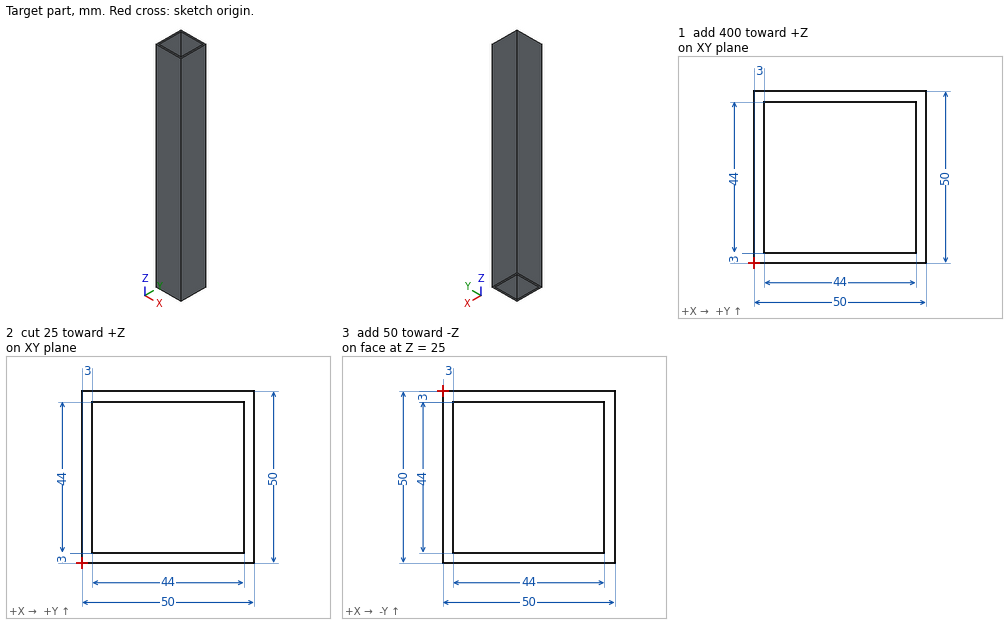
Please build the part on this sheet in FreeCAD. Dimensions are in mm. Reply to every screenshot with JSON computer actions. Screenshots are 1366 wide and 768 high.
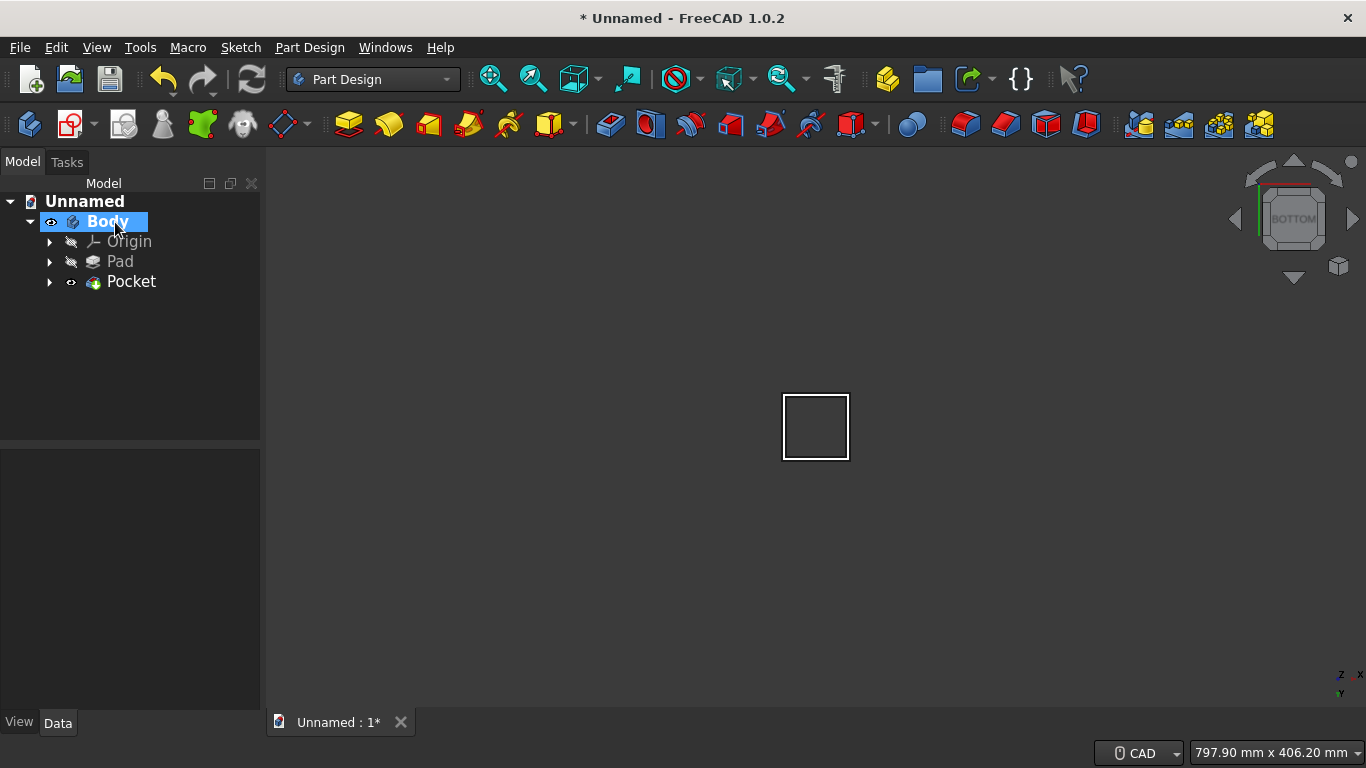
{"action": "left_click", "coordinate": [494, 80]}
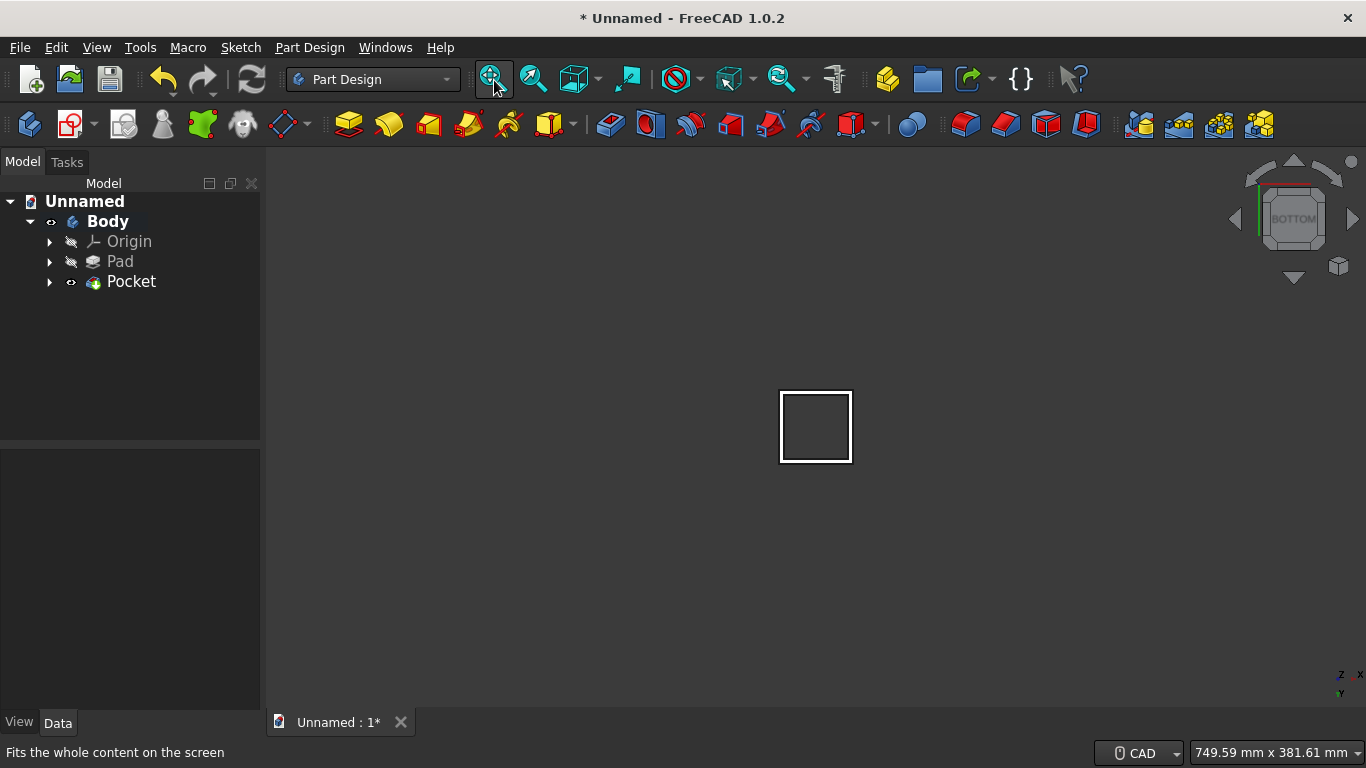
{"action": "scroll", "coordinate": [851, 415], "scroll_direction": "up", "scroll_amount": 11}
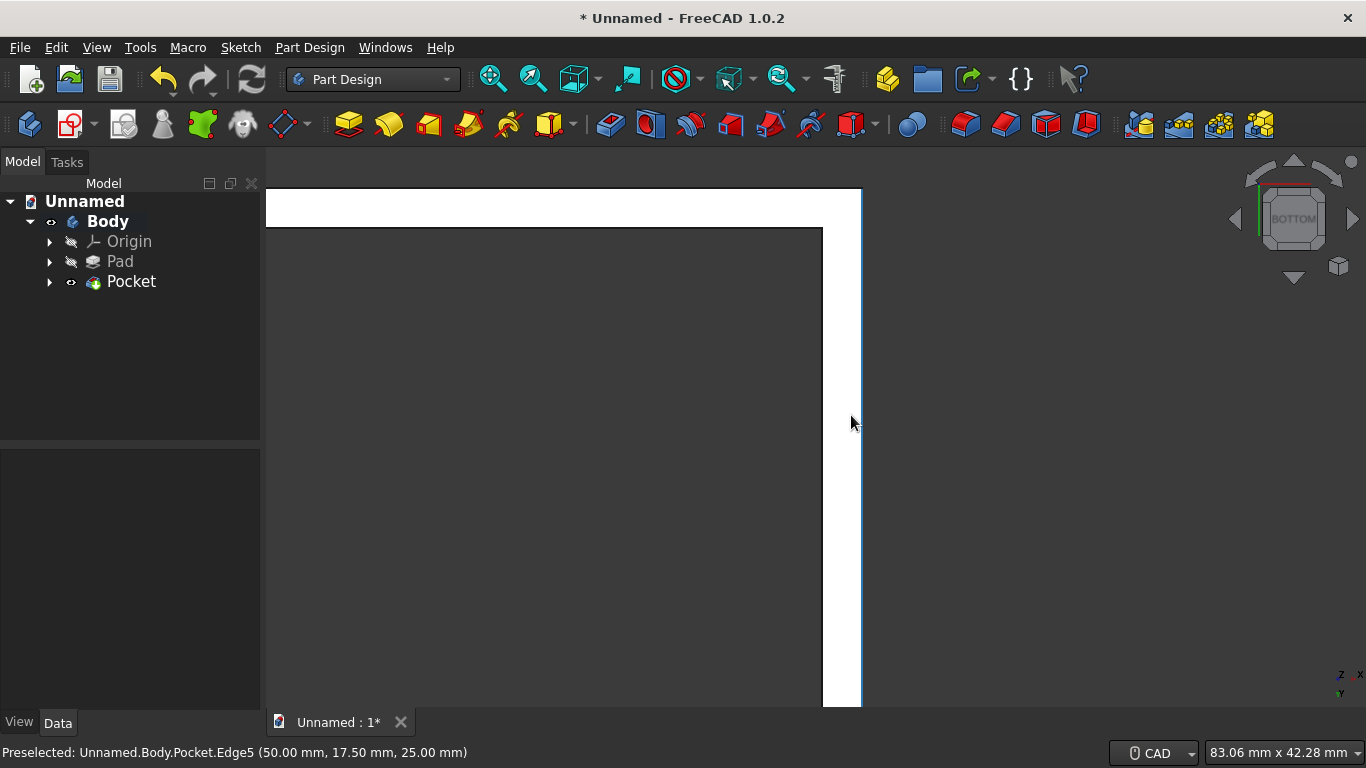
{"action": "left_click", "coordinate": [849, 421]}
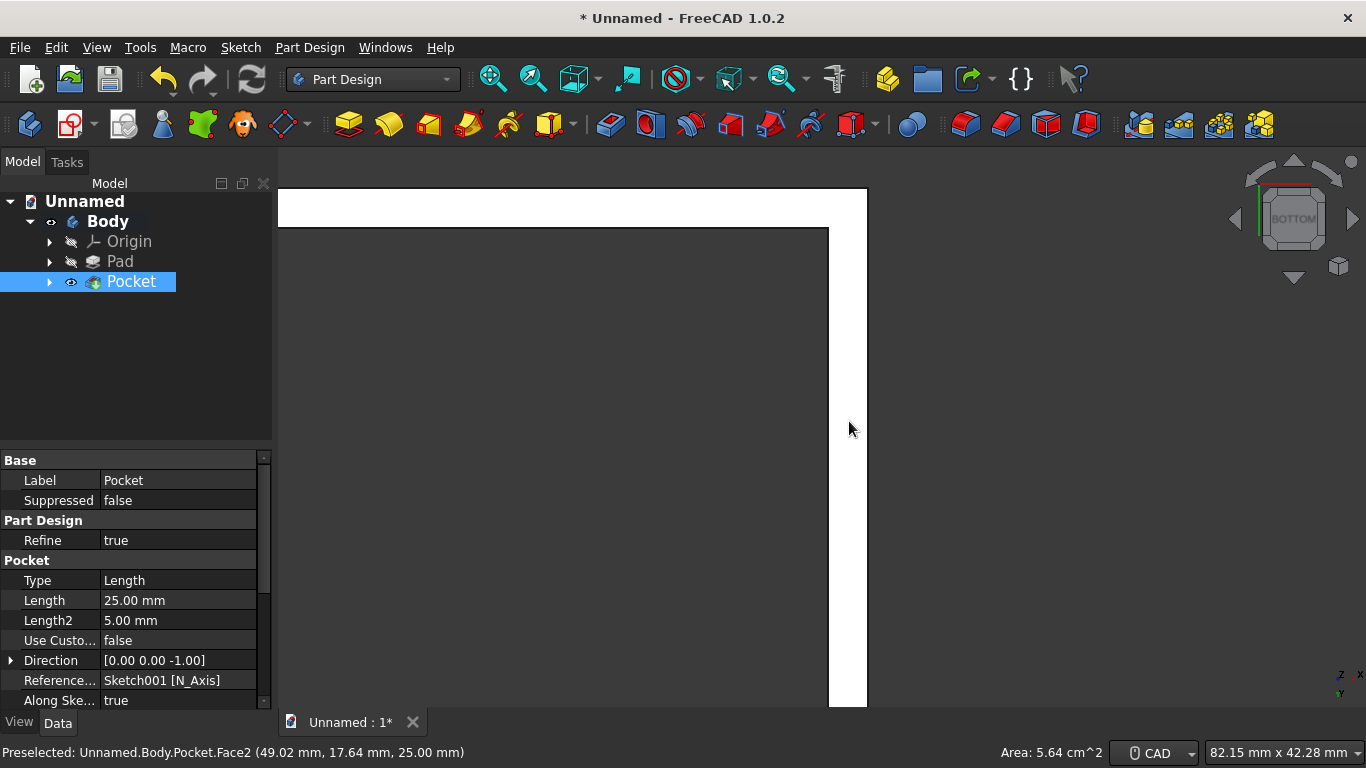
{"action": "left_click", "coordinate": [70, 124]}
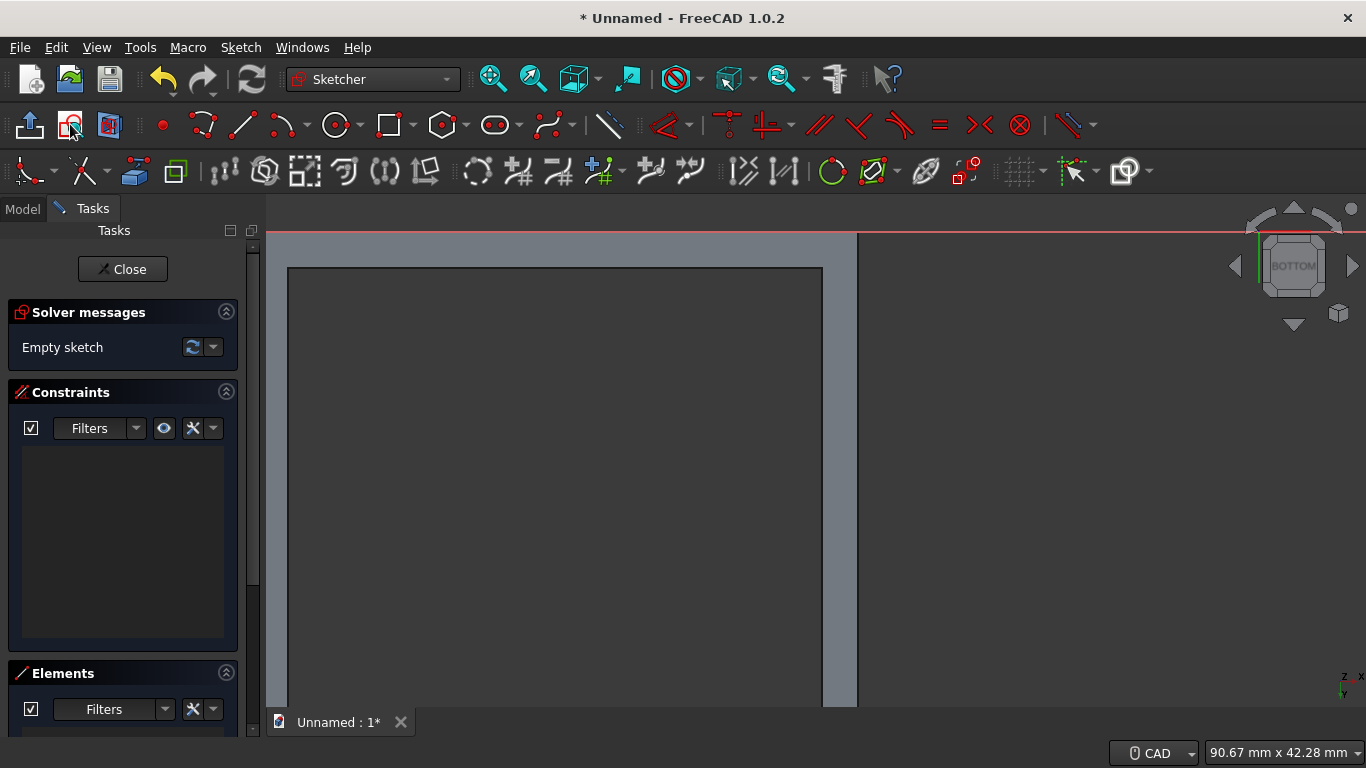
{"action": "scroll", "coordinate": [982, 347], "scroll_direction": "down", "scroll_amount": 3}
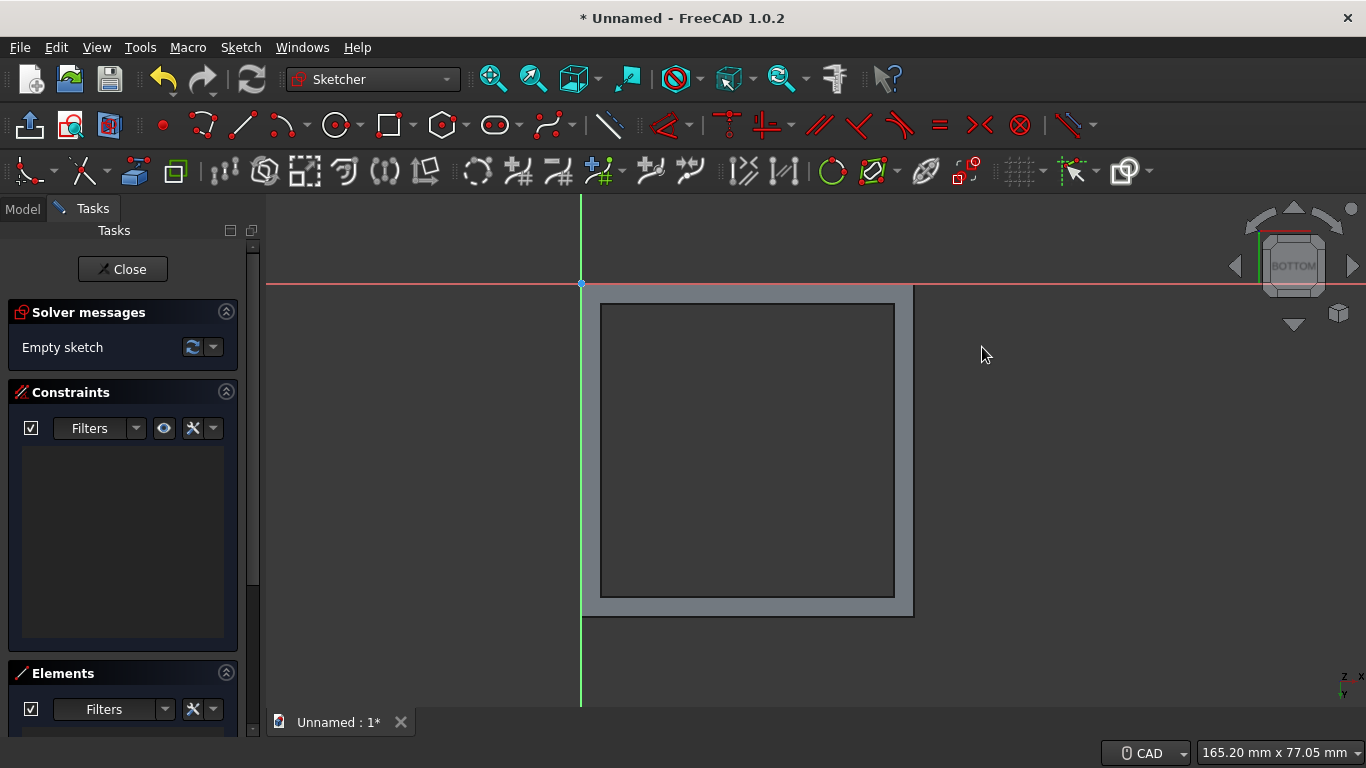
{"action": "left_click", "coordinate": [390, 126]}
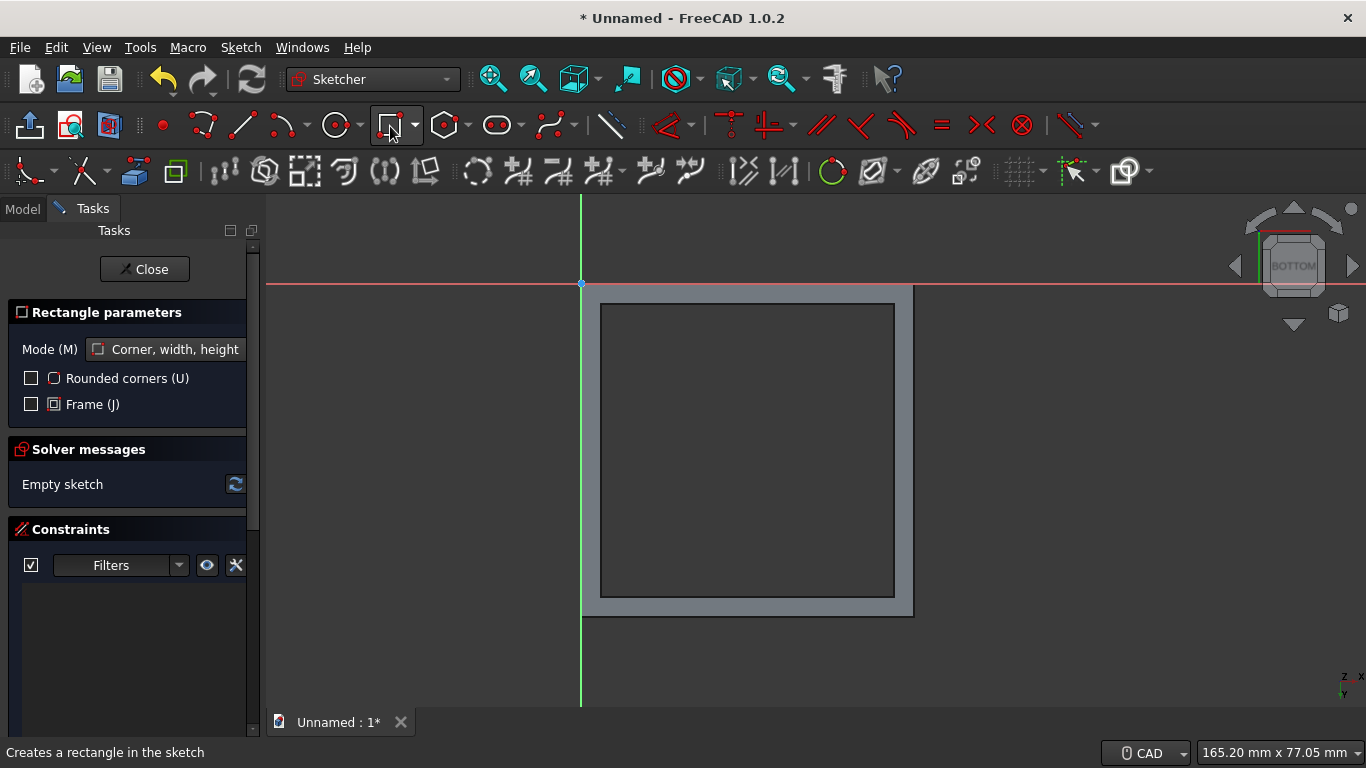
{"action": "left_click", "coordinate": [581, 284]}
{"action": "left_click", "coordinate": [914, 617]}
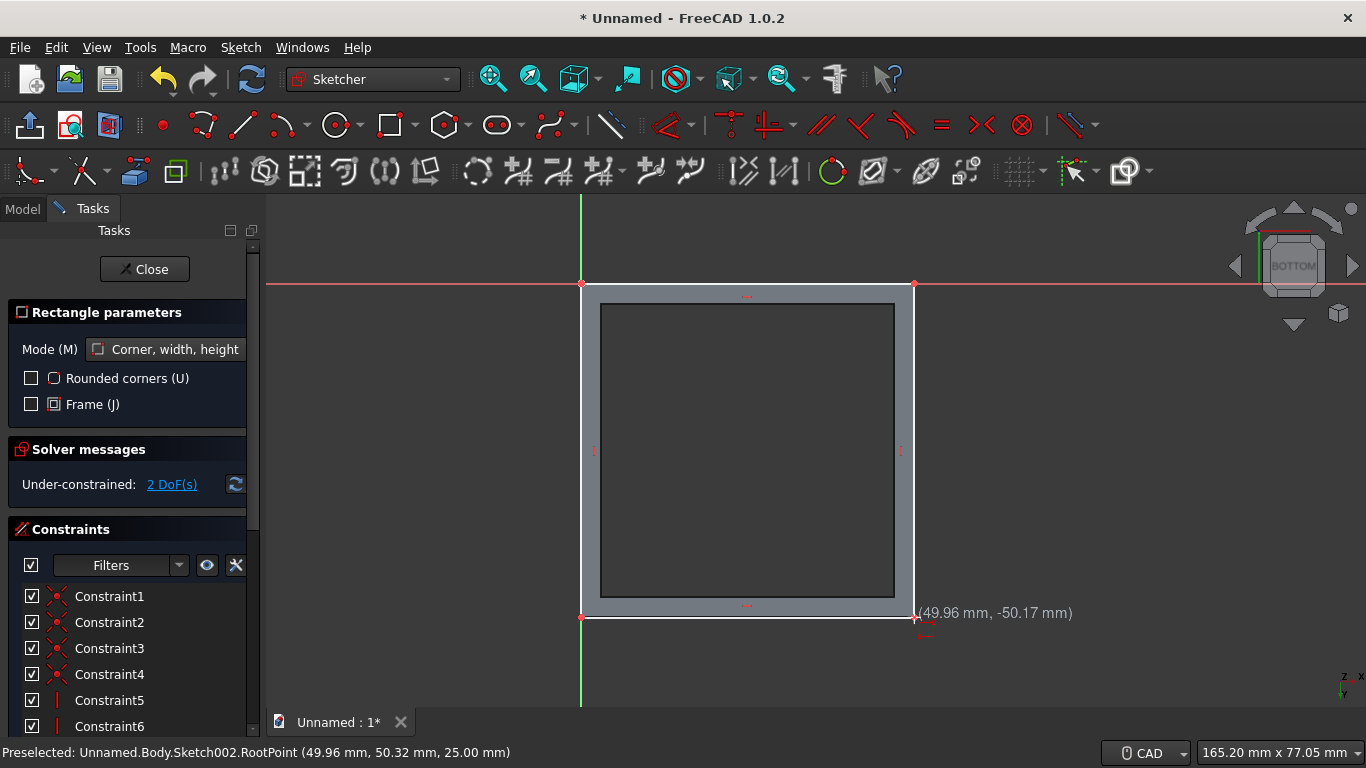
{"action": "left_click", "coordinate": [601, 304]}
{"action": "left_click", "coordinate": [894, 597]}
{"action": "key", "text": "Escape"}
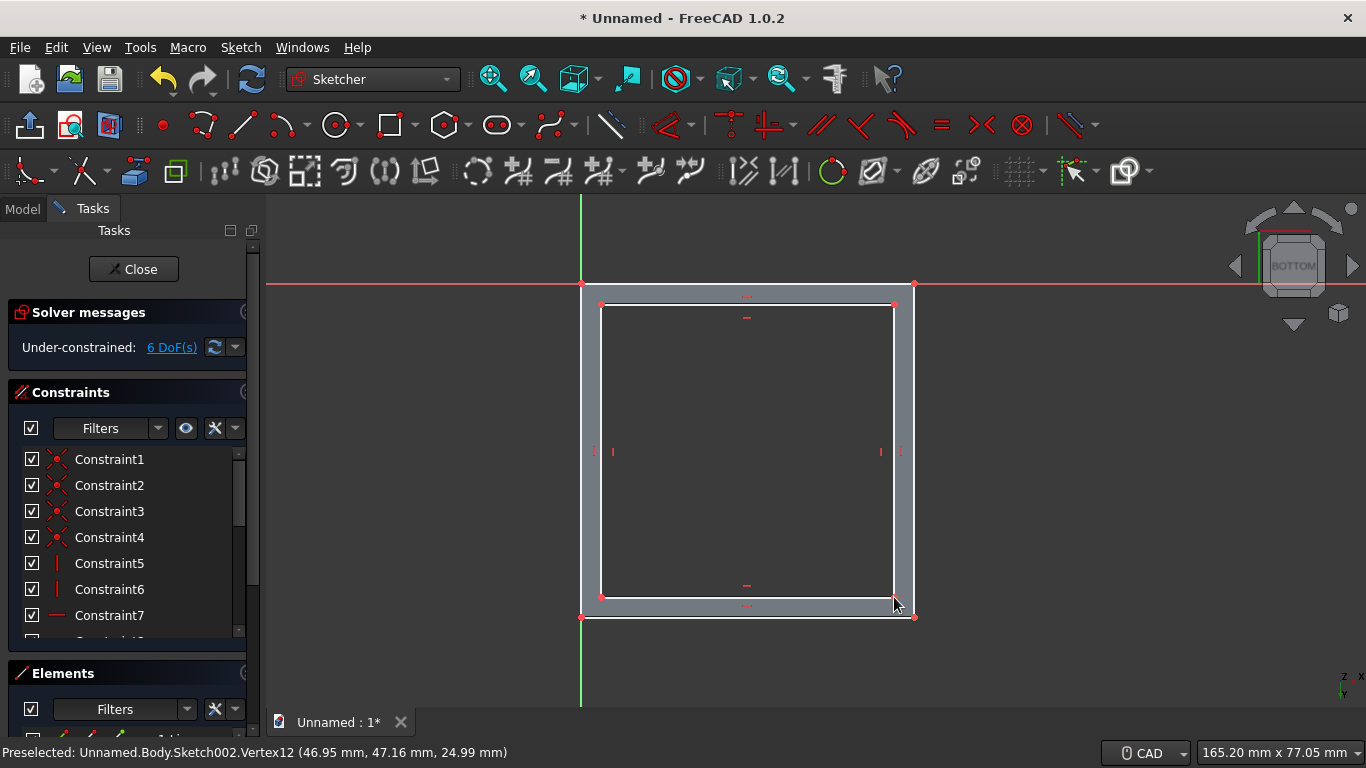
{"action": "left_click", "coordinate": [666, 126]}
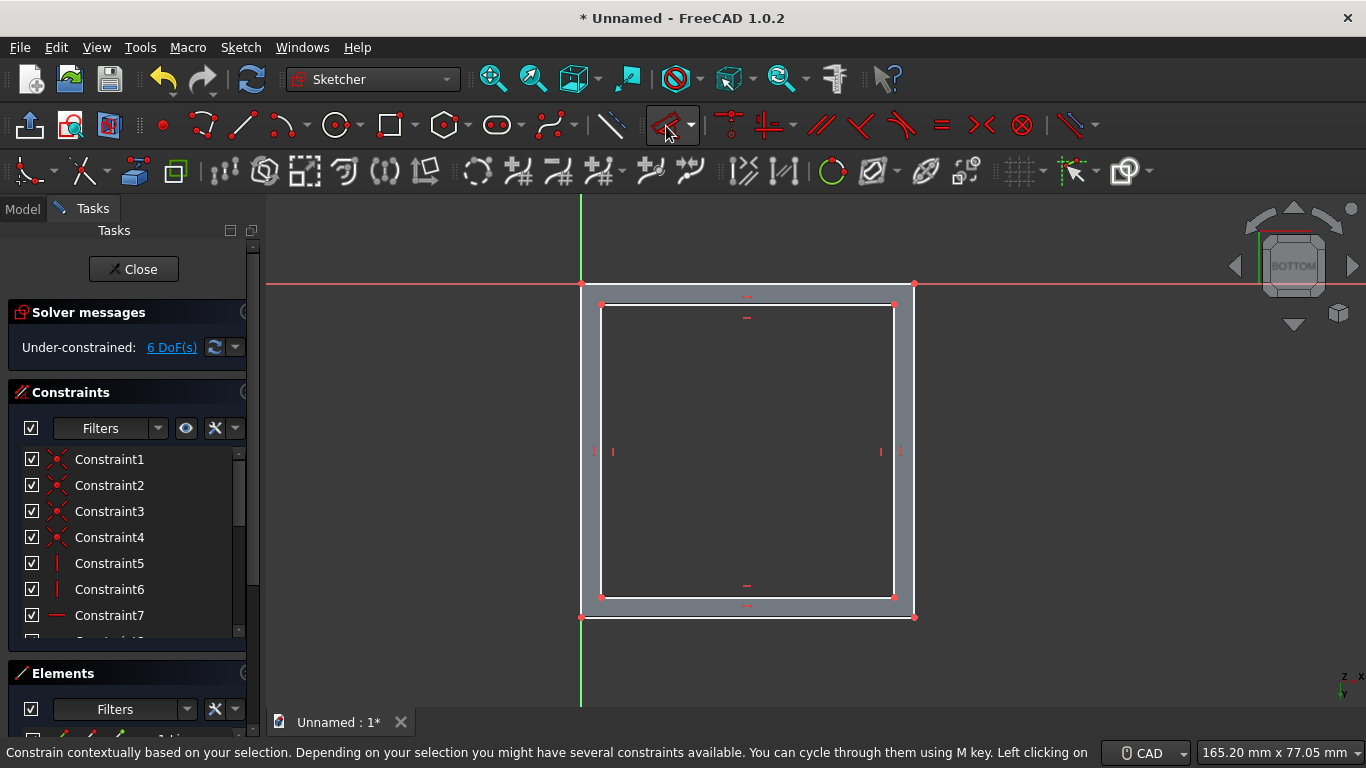
{"action": "left_click", "coordinate": [581, 384]}
{"action": "left_click", "coordinate": [547, 451]}